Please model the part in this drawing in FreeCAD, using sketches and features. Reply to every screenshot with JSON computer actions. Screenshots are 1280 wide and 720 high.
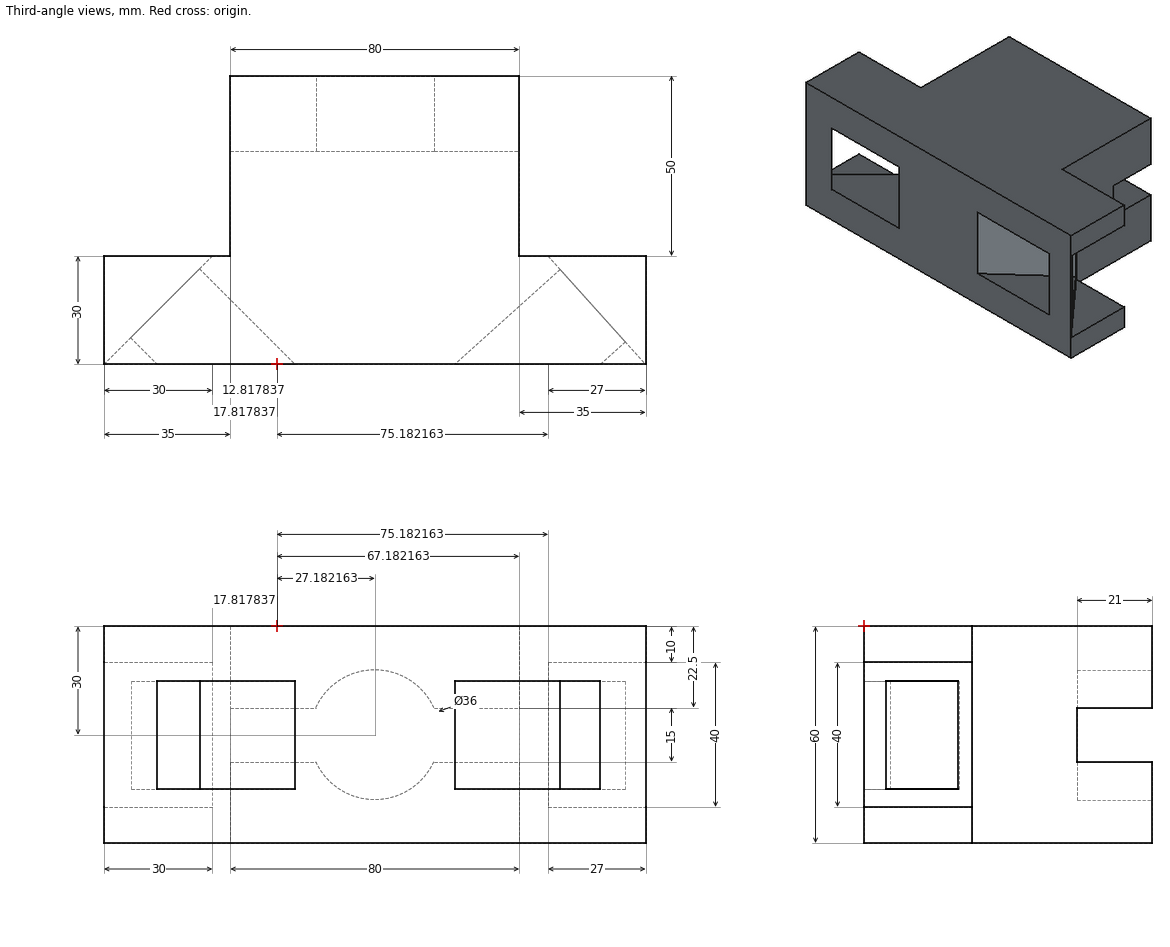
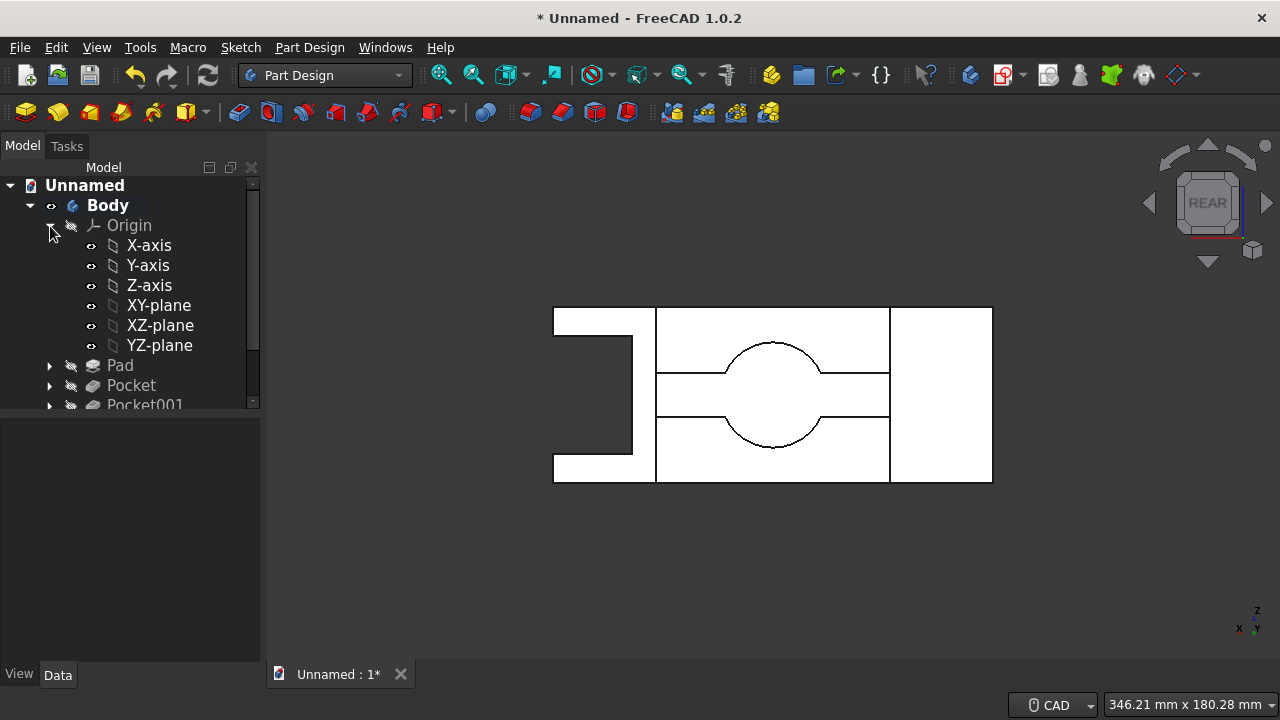
{"action": "left_click", "coordinate": [136, 306]}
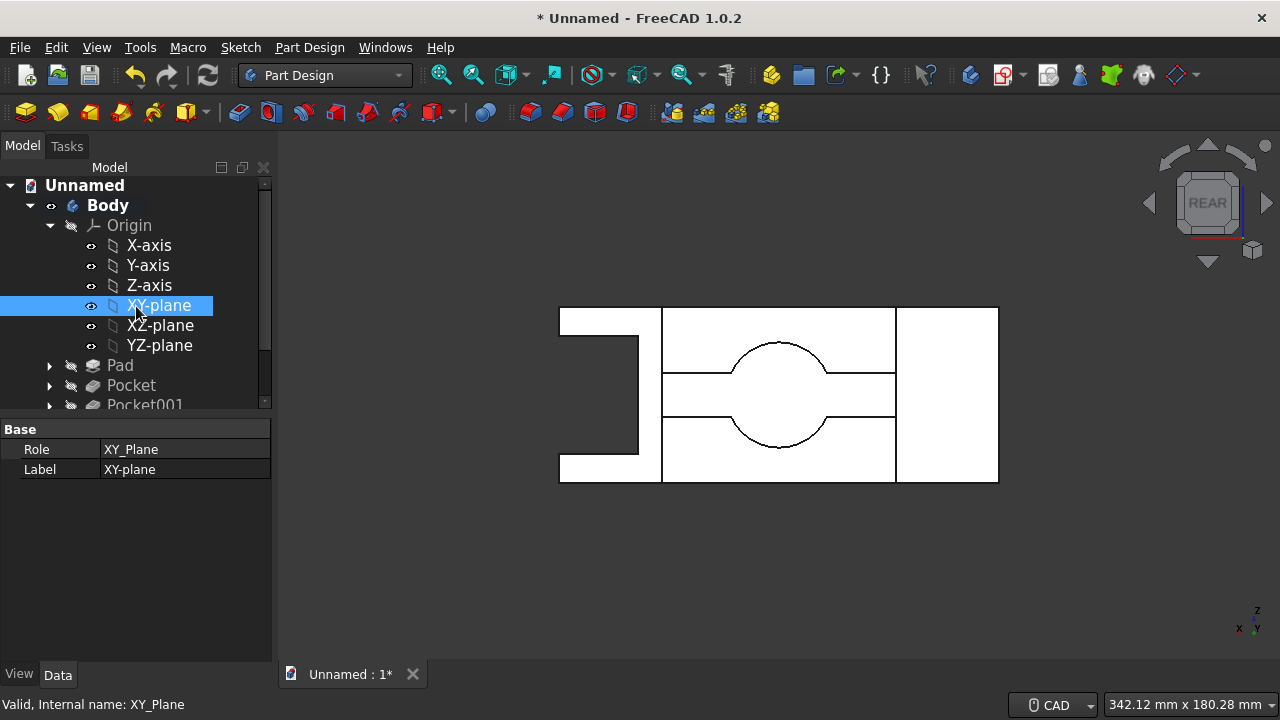
{"action": "left_click", "coordinate": [1176, 76]}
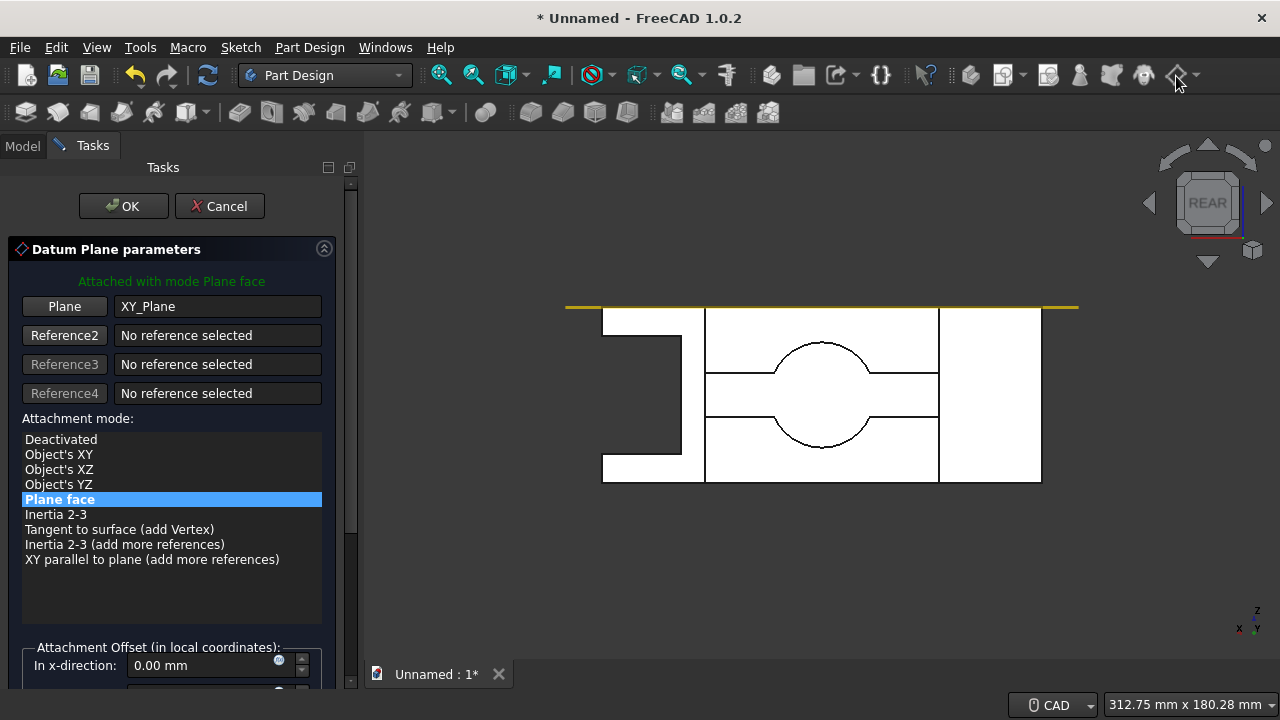
{"action": "scroll", "coordinate": [351, 432], "scroll_direction": "down", "scroll_amount": 2}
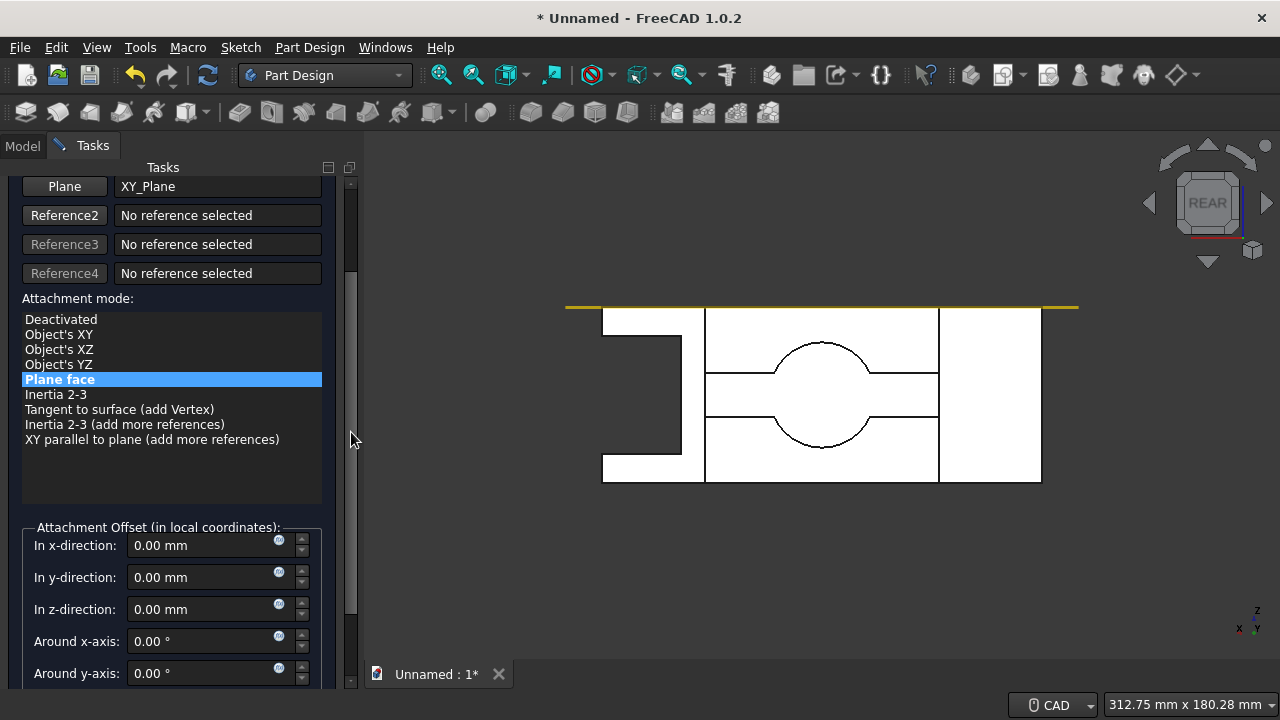
{"action": "triple_click", "coordinate": [210, 609]}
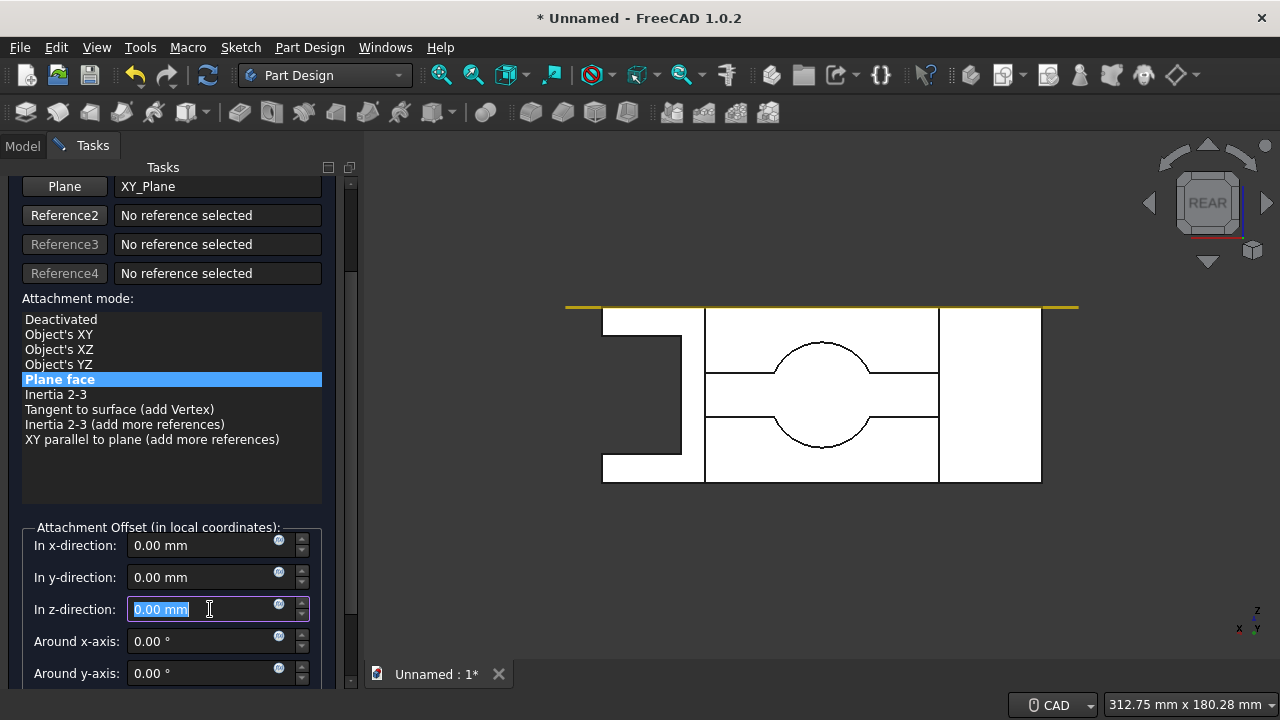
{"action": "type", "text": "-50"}
{"action": "key", "text": "Tab"}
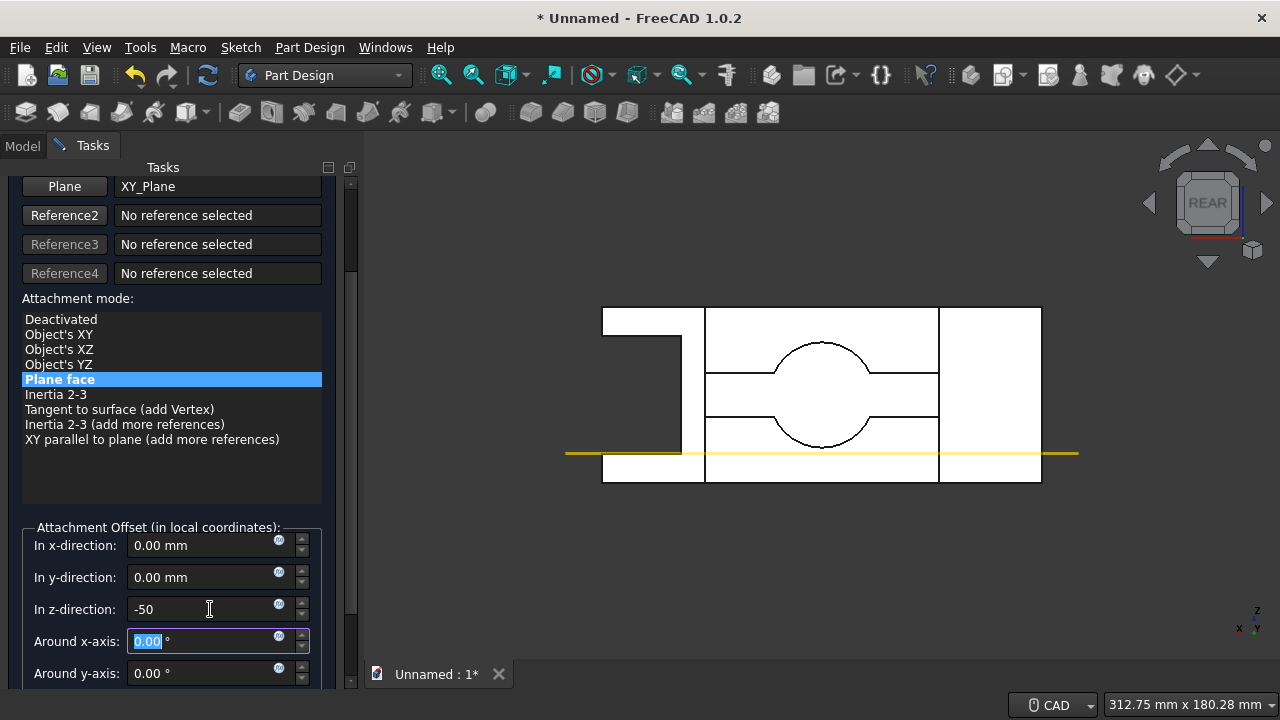
{"action": "scroll", "coordinate": [351, 432], "scroll_direction": "up", "scroll_amount": 3}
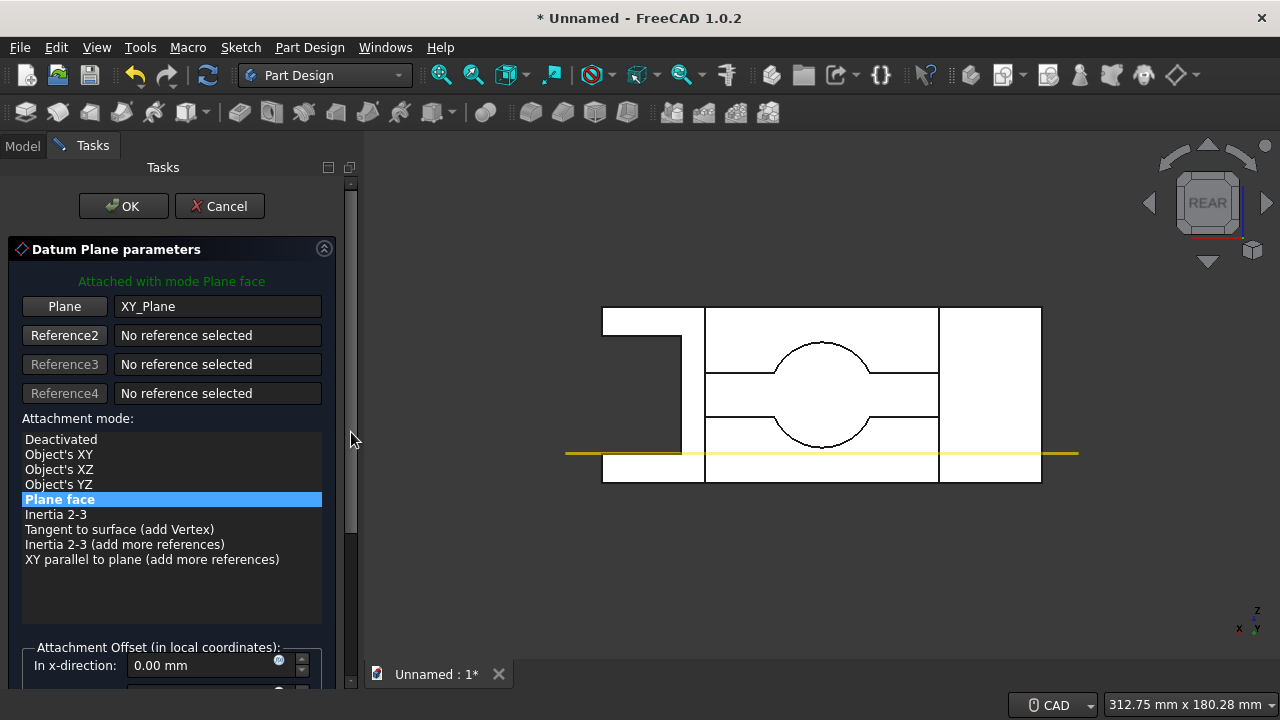
{"action": "left_click", "coordinate": [124, 206]}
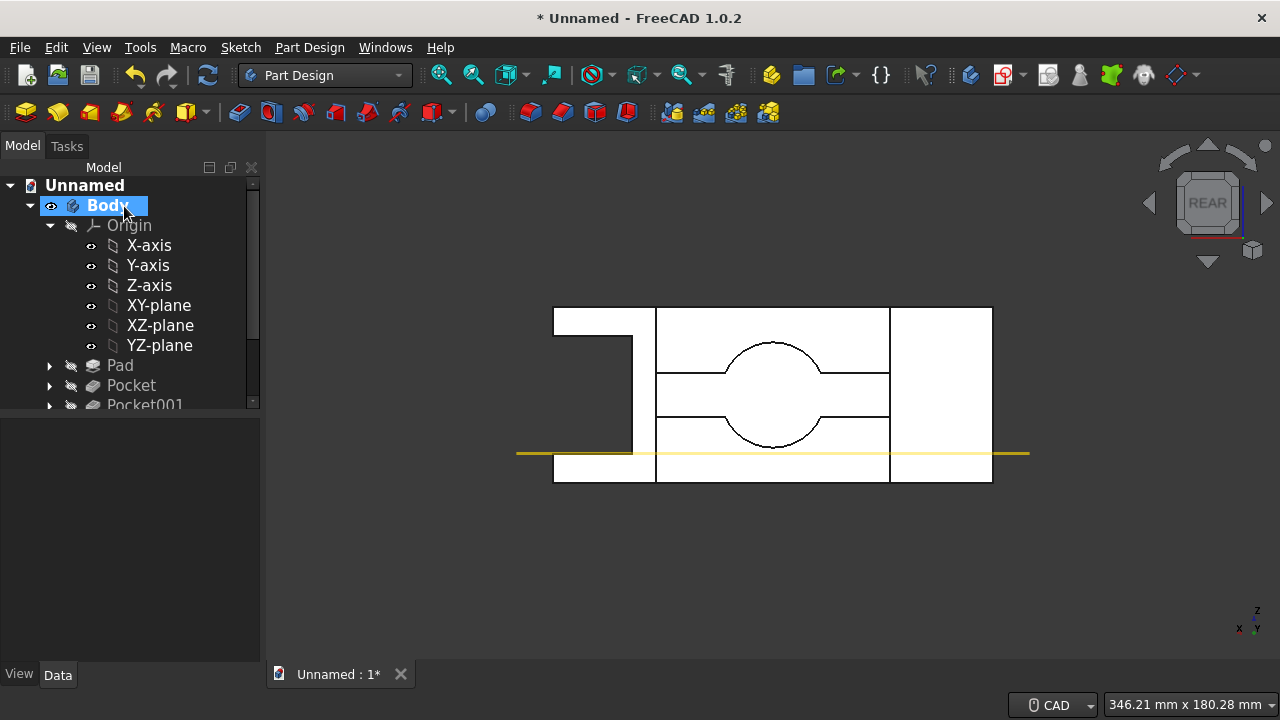
{"action": "scroll", "coordinate": [100, 301], "scroll_direction": "down", "scroll_amount": 3}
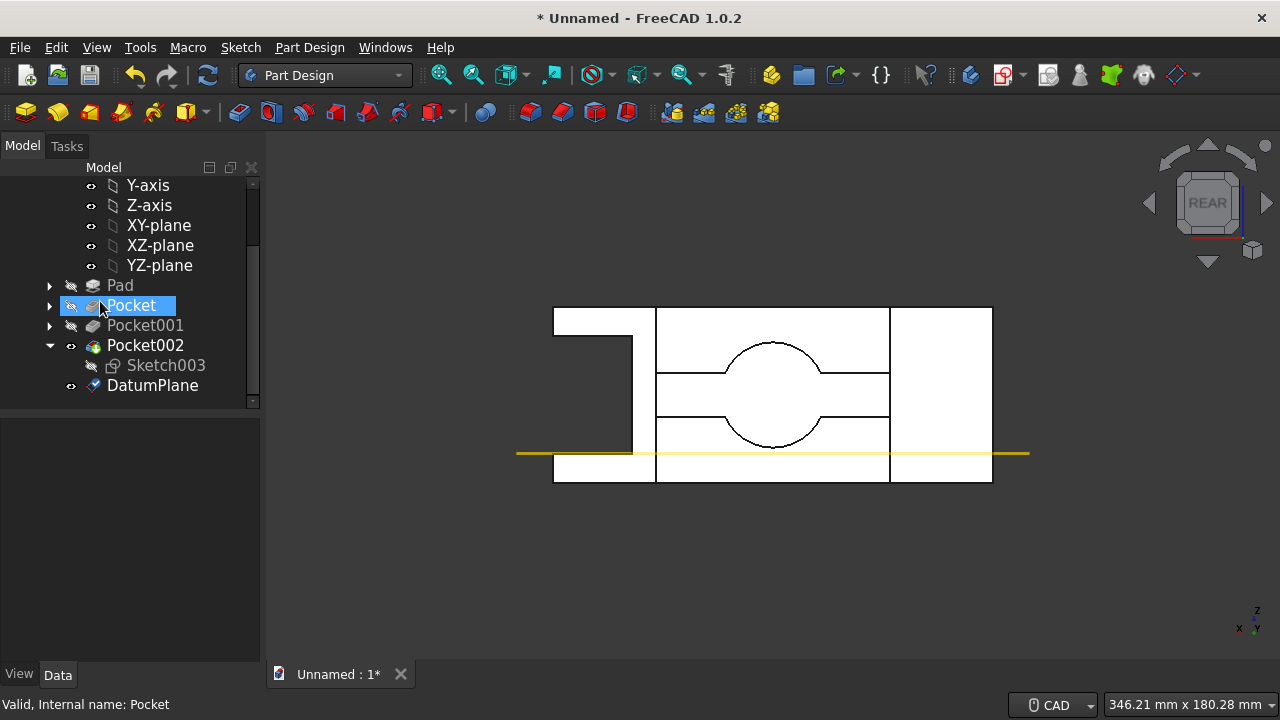
{"action": "left_click", "coordinate": [116, 386]}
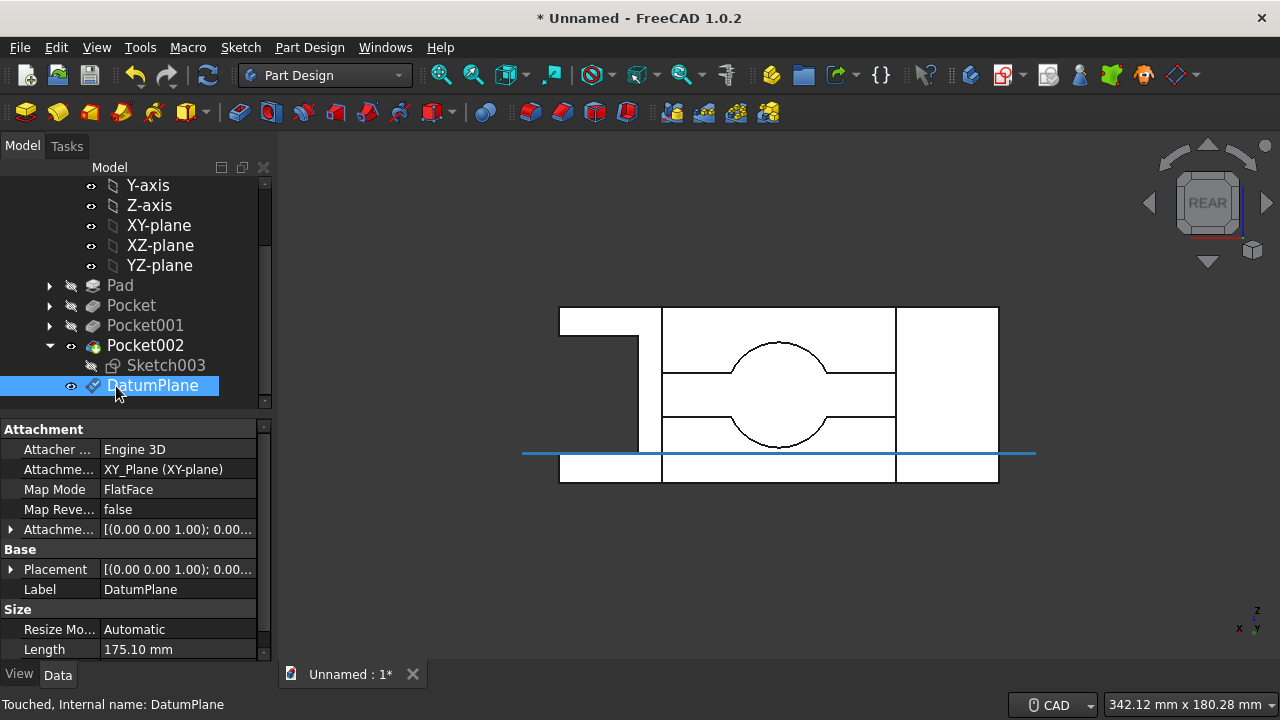
{"action": "left_click", "coordinate": [1004, 76]}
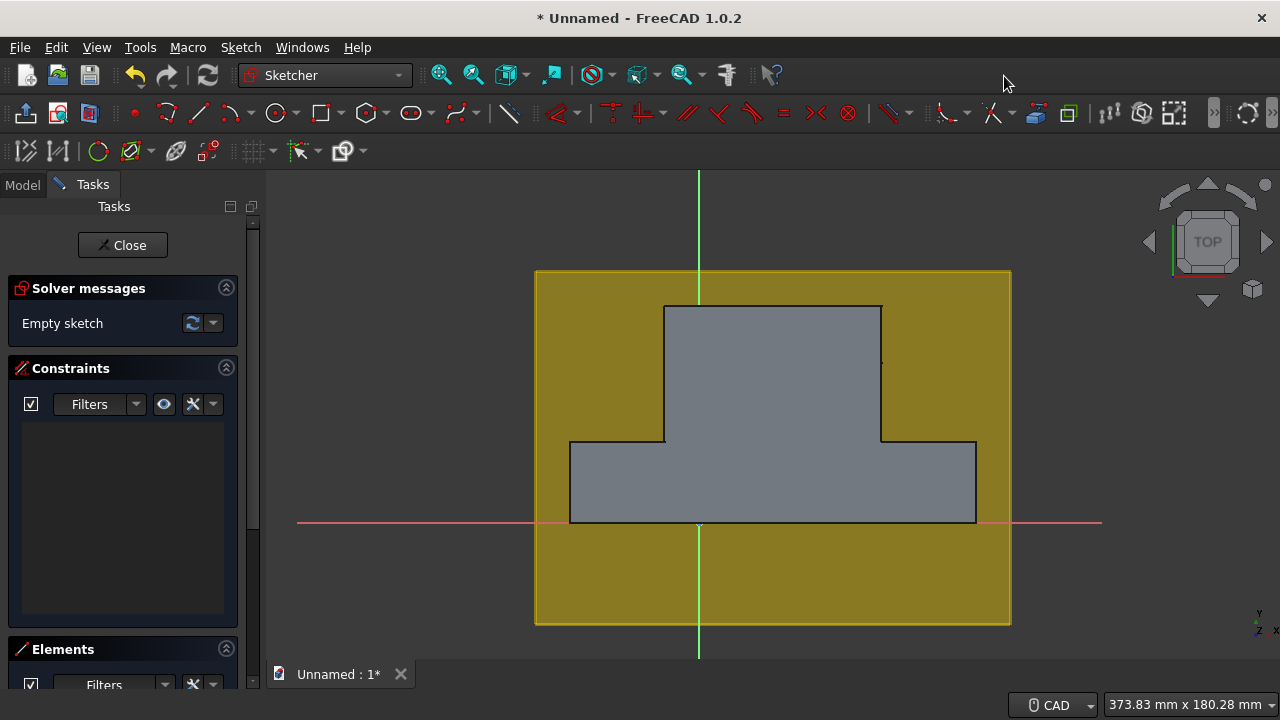
{"action": "left_click", "coordinate": [90, 114]}